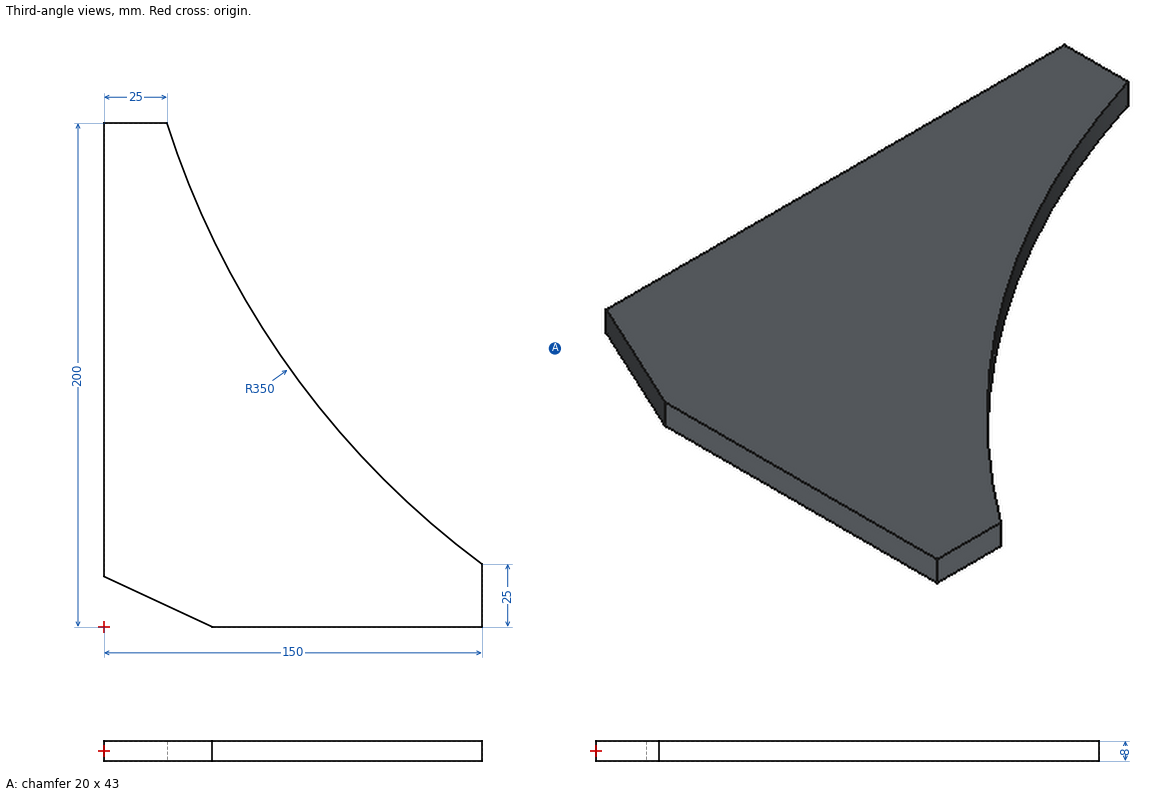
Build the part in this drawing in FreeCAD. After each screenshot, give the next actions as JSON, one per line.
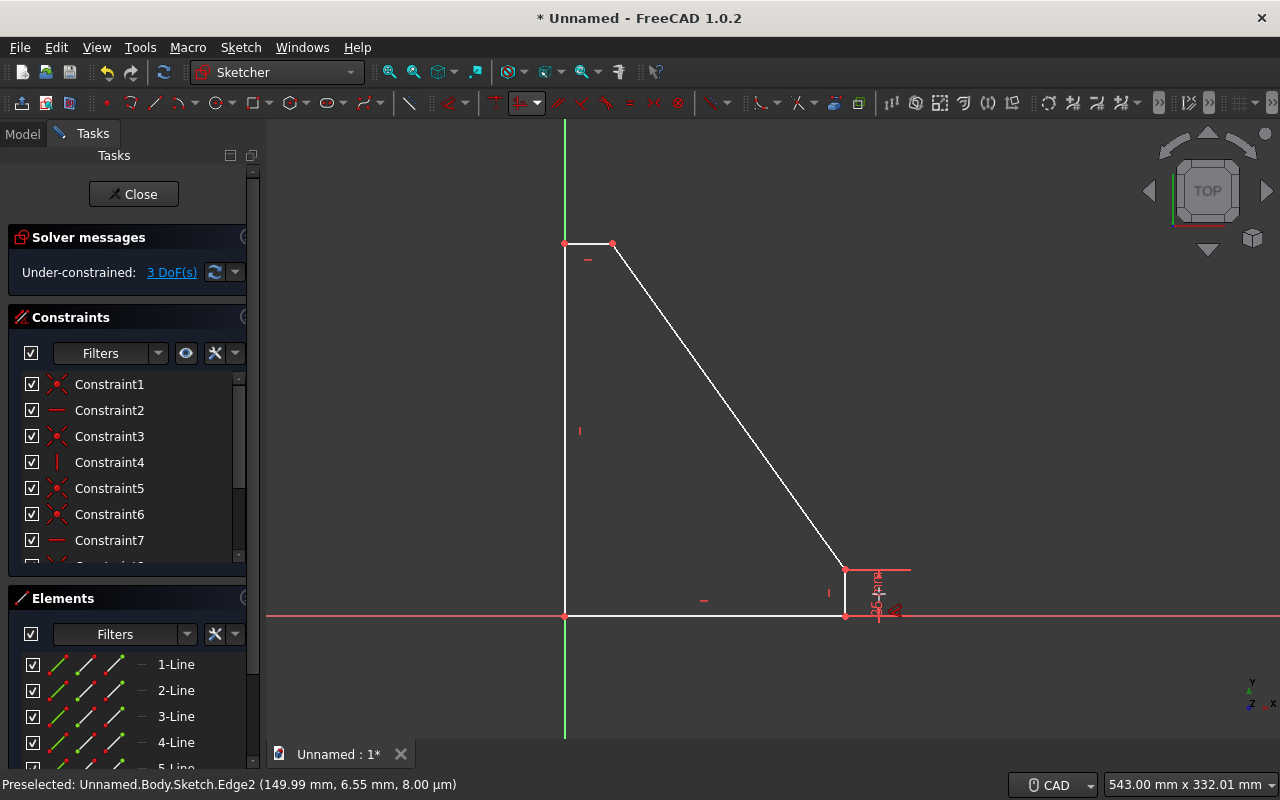
{"action": "left_click", "coordinate": [598, 244]}
{"action": "left_click", "coordinate": [588, 210]}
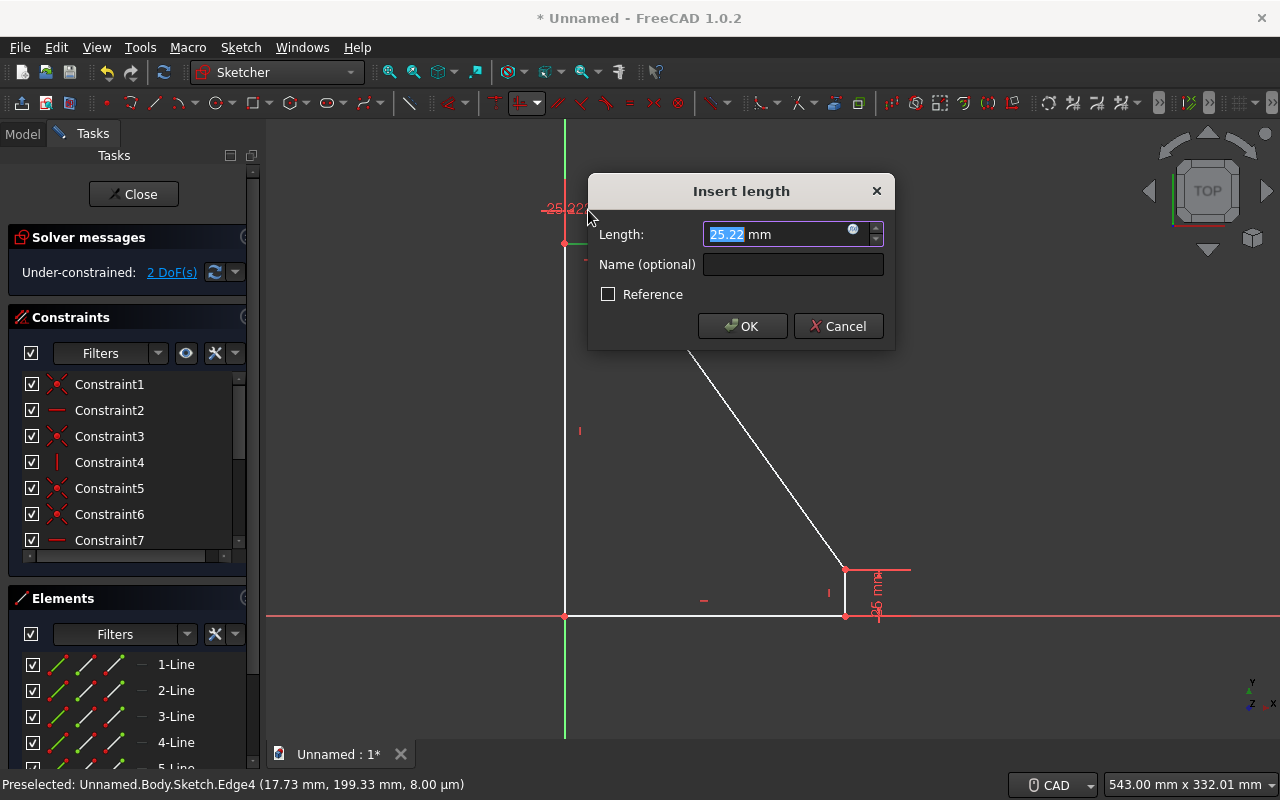
{"action": "type", "text": "25"}
{"action": "key", "text": "Return"}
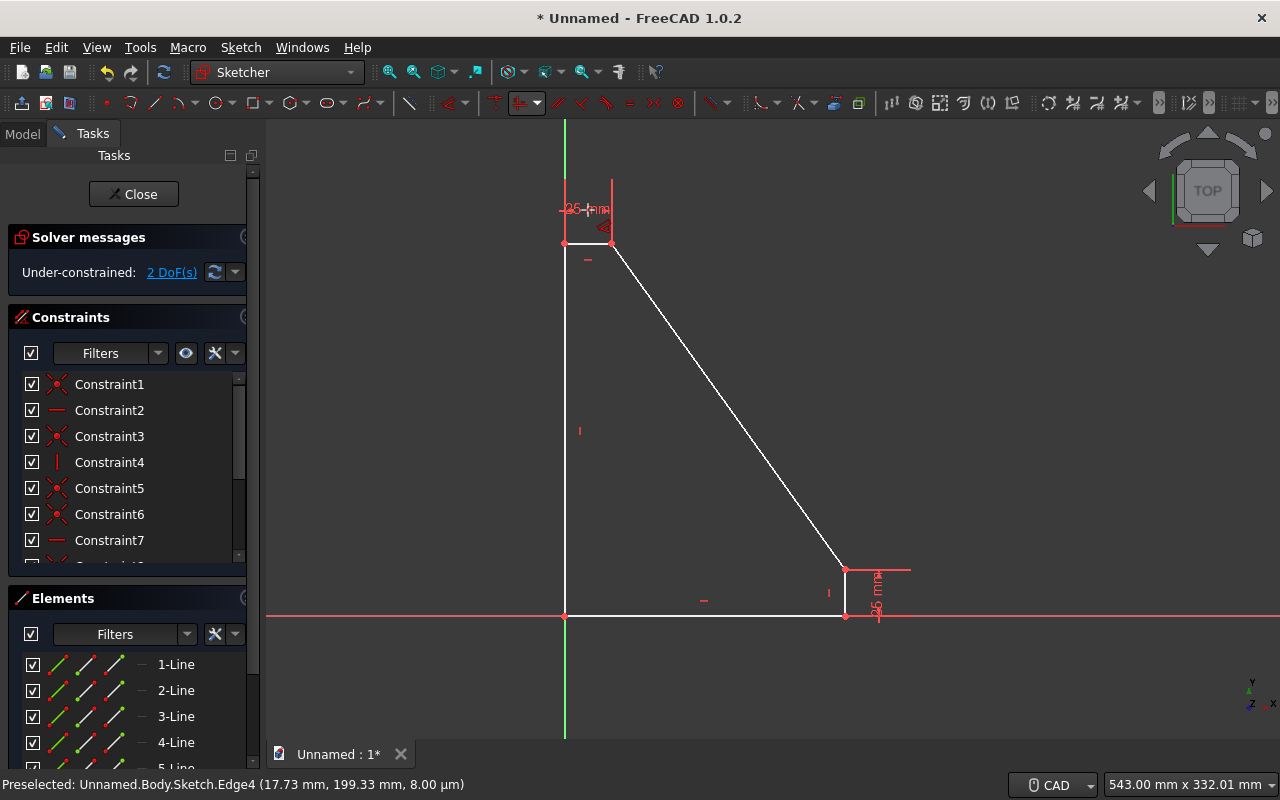
{"action": "left_click", "coordinate": [649, 616]}
{"action": "left_click", "coordinate": [705, 650]}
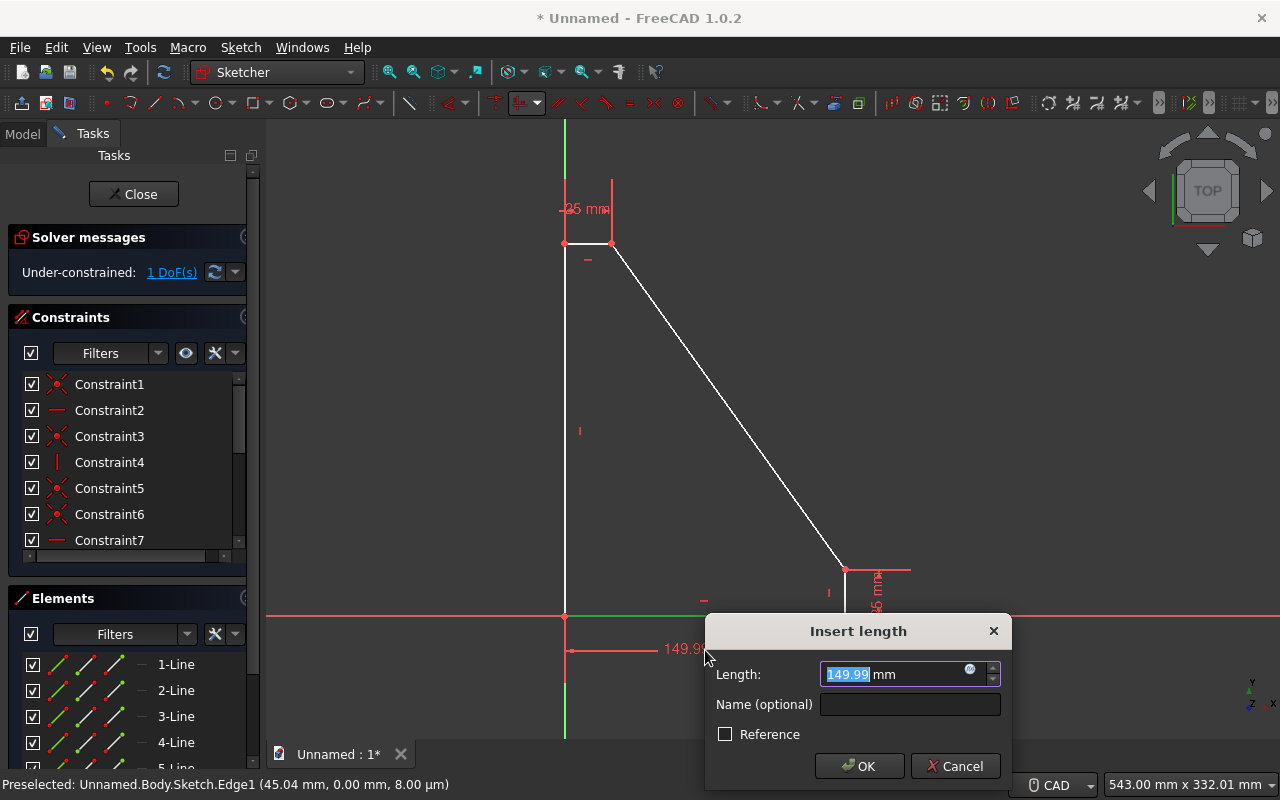
{"action": "type", "text": "150"}
{"action": "key", "text": "Return"}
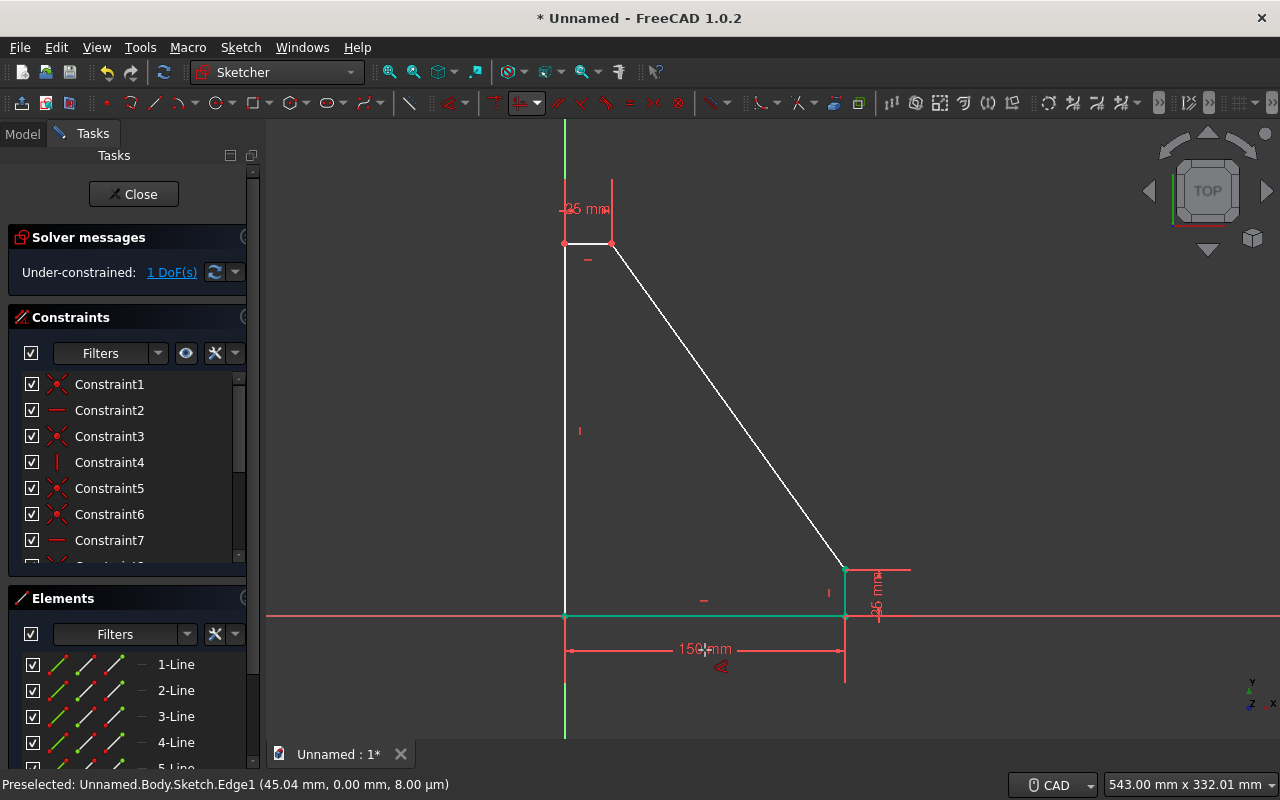
{"action": "left_click", "coordinate": [565, 356]}
{"action": "left_click", "coordinate": [531, 430]}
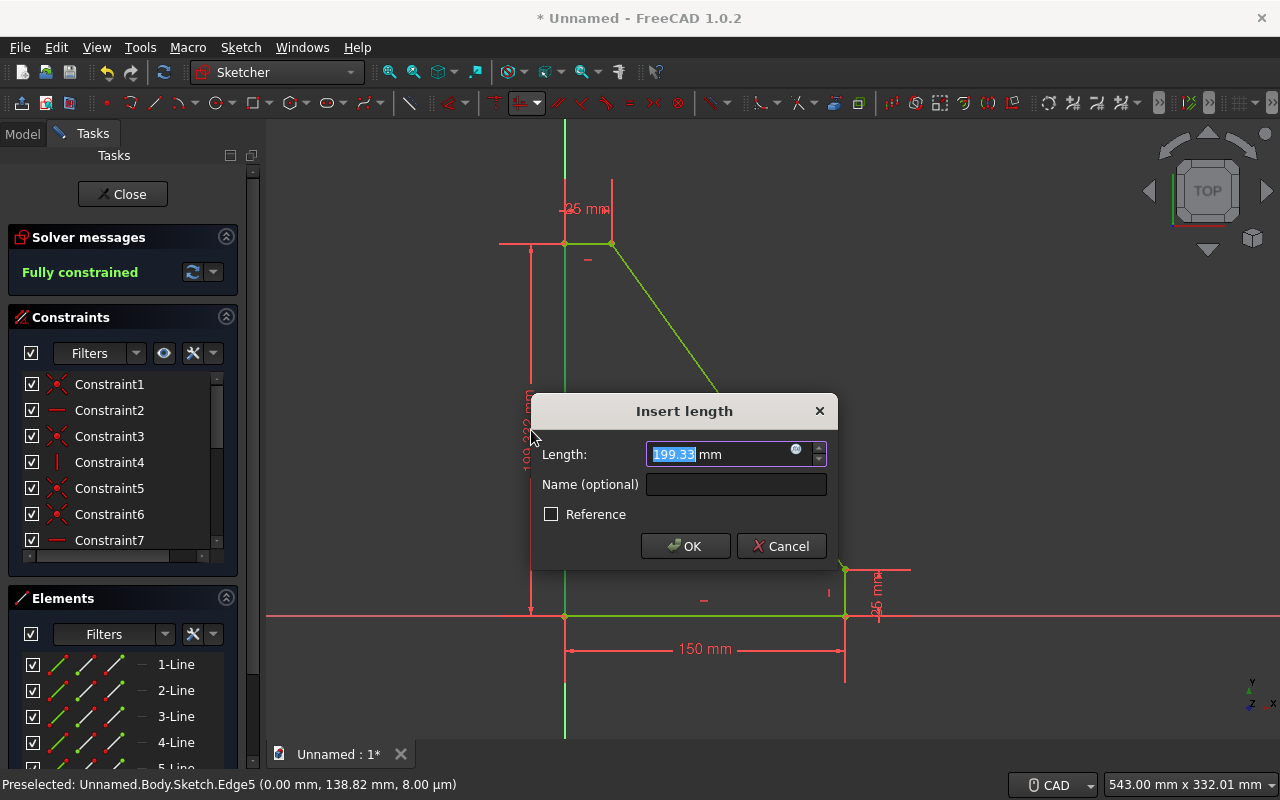
{"action": "type", "text": "200"}
{"action": "key", "text": "Return"}
{"action": "key", "text": "Escape"}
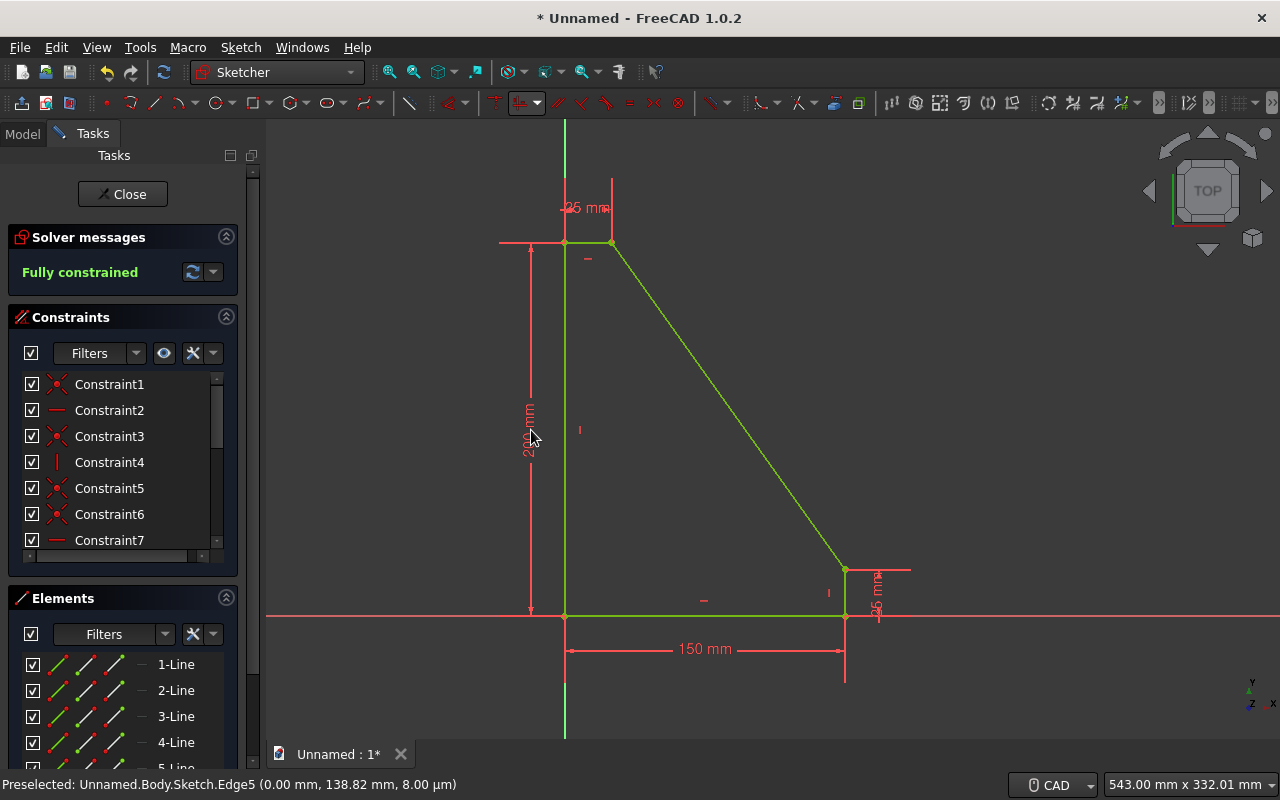
{"action": "left_click", "coordinate": [123, 194]}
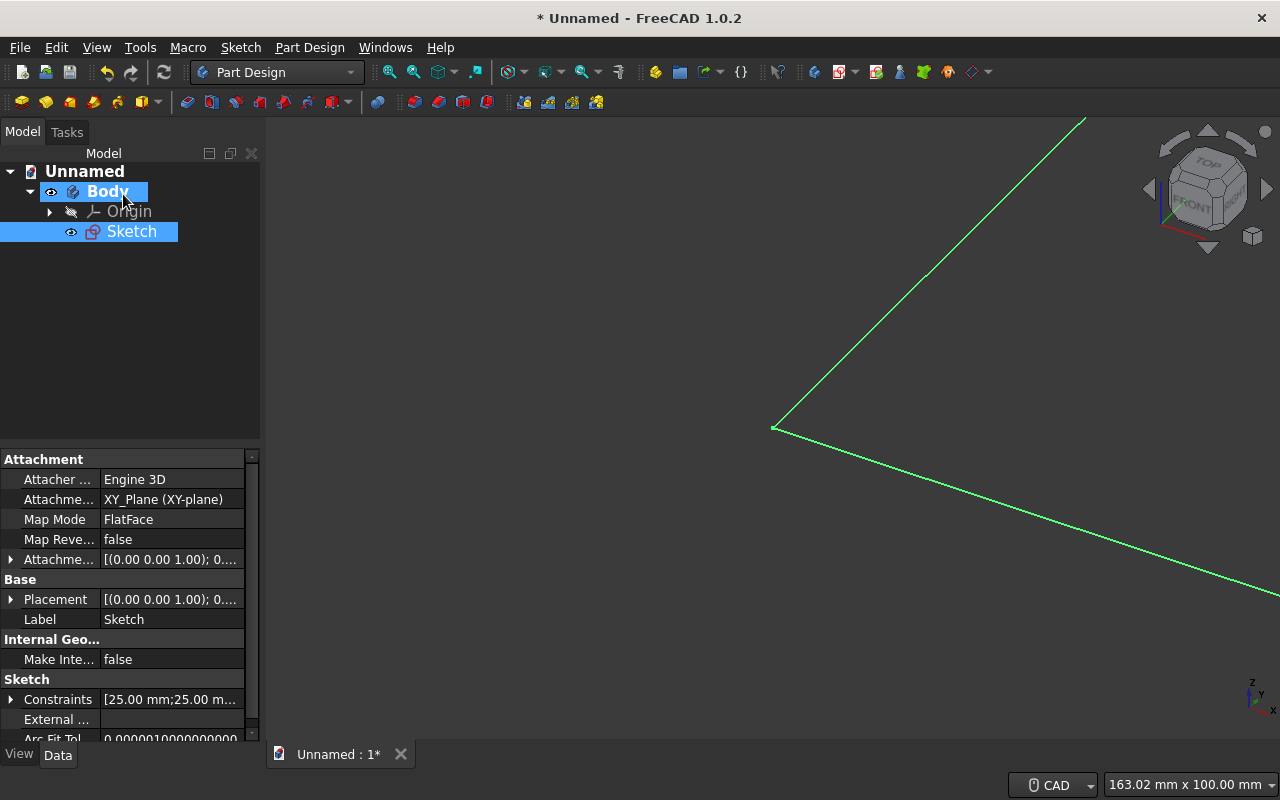
{"action": "left_click", "coordinate": [22, 102]}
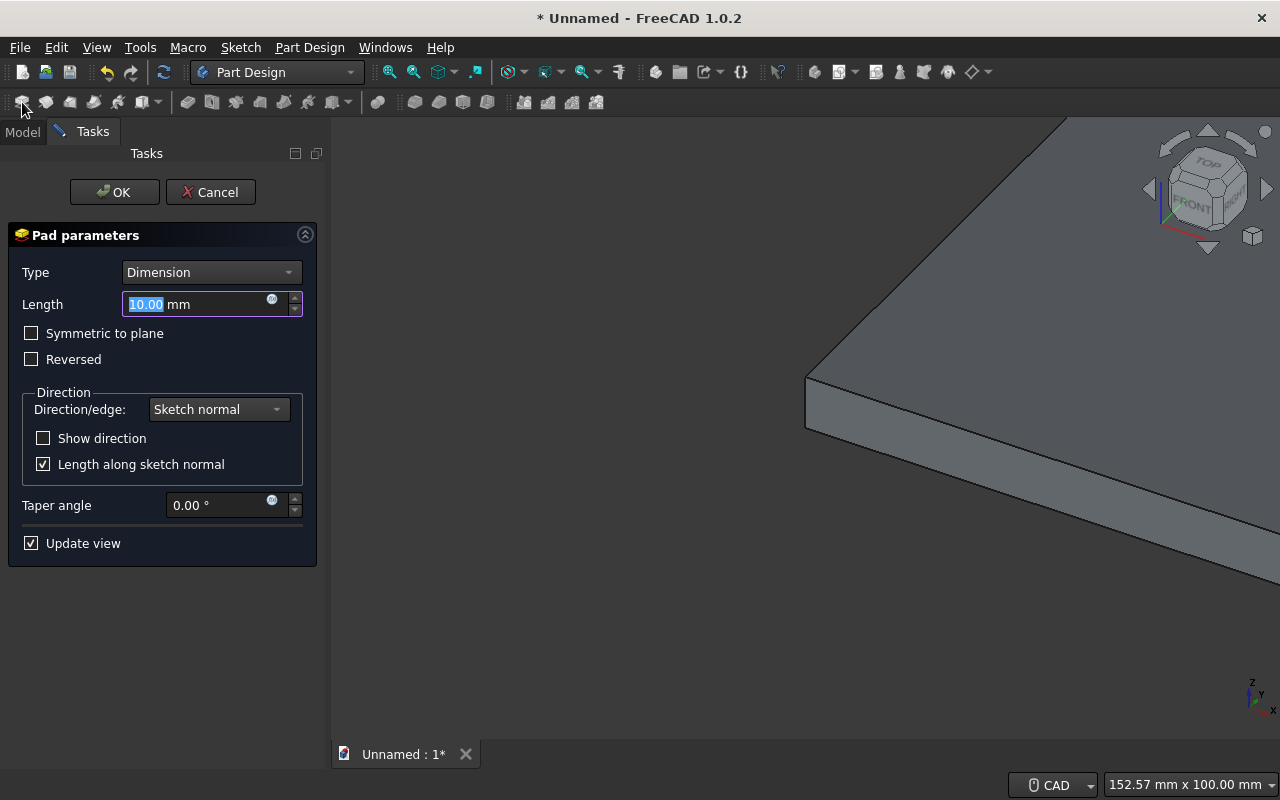
{"action": "type", "text": "8"}
{"action": "key", "text": "Tab"}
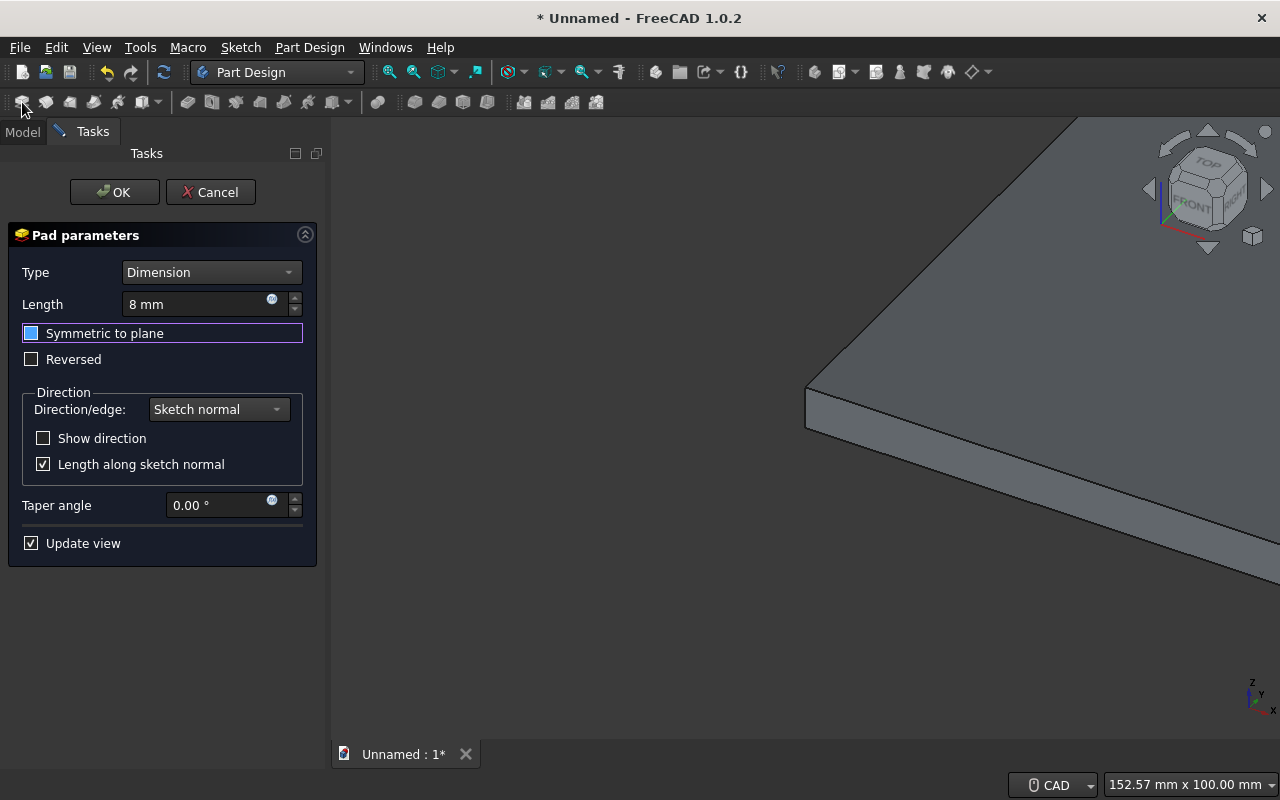
{"action": "left_click", "coordinate": [30, 333]}